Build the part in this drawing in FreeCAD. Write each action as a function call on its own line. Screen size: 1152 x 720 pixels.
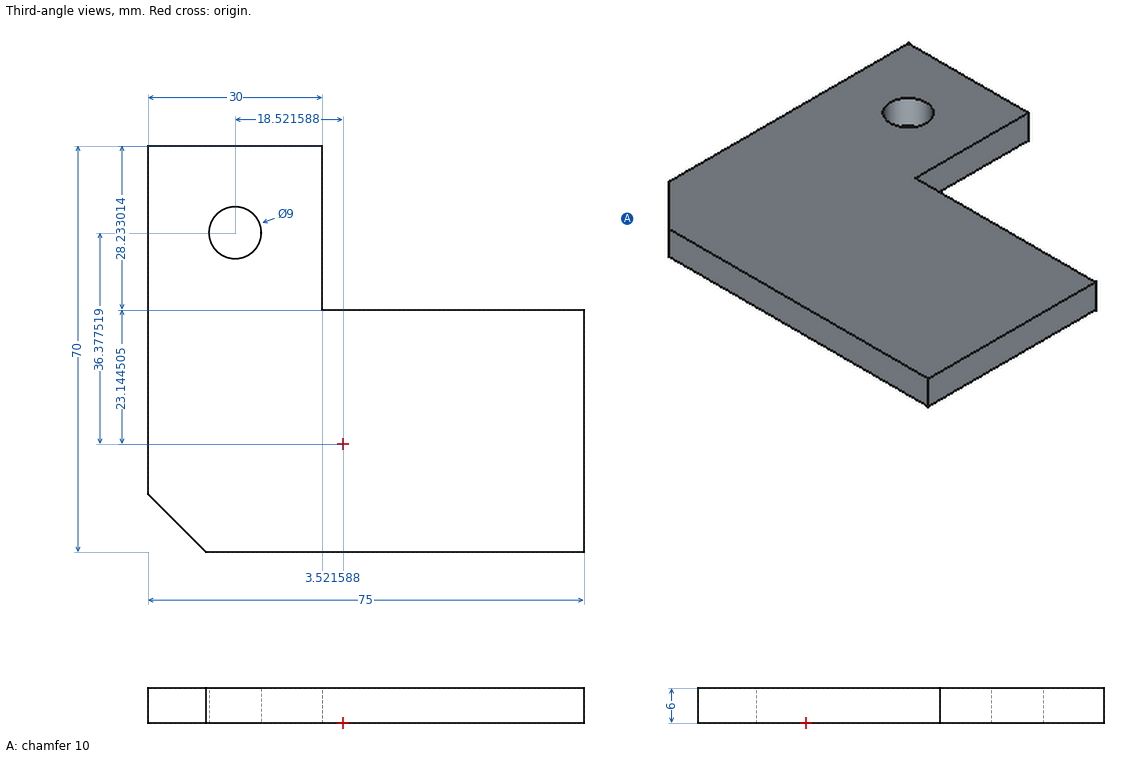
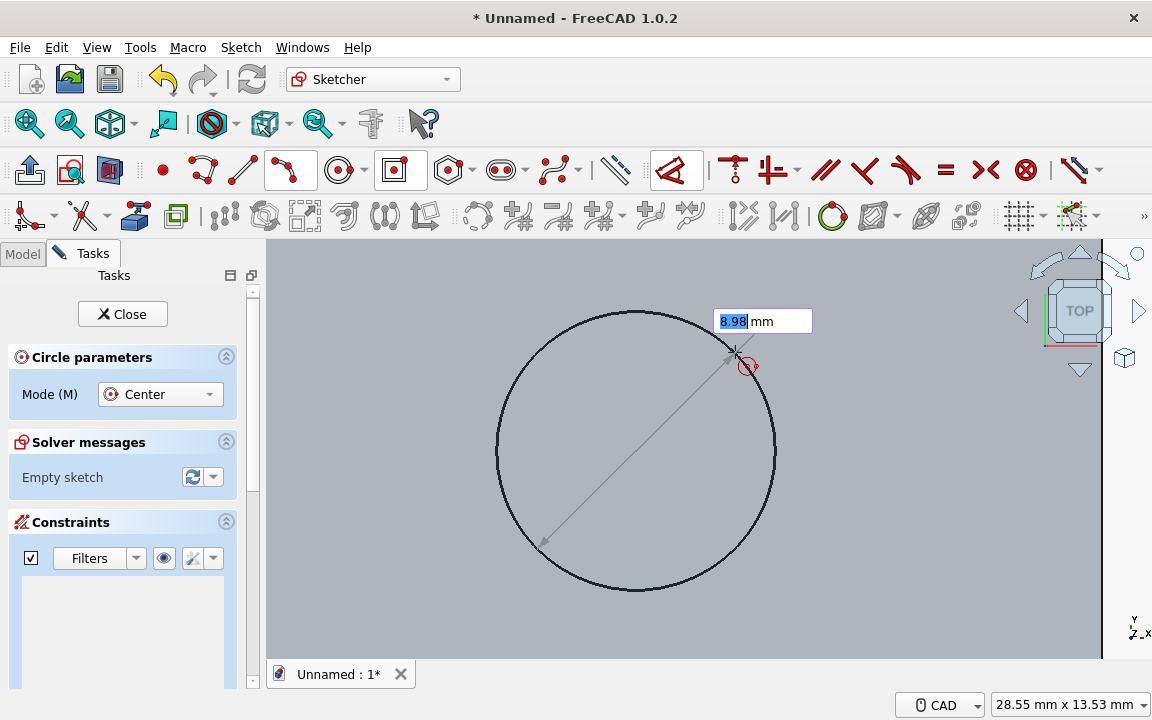
text(9)
key(Return)
key(Escape)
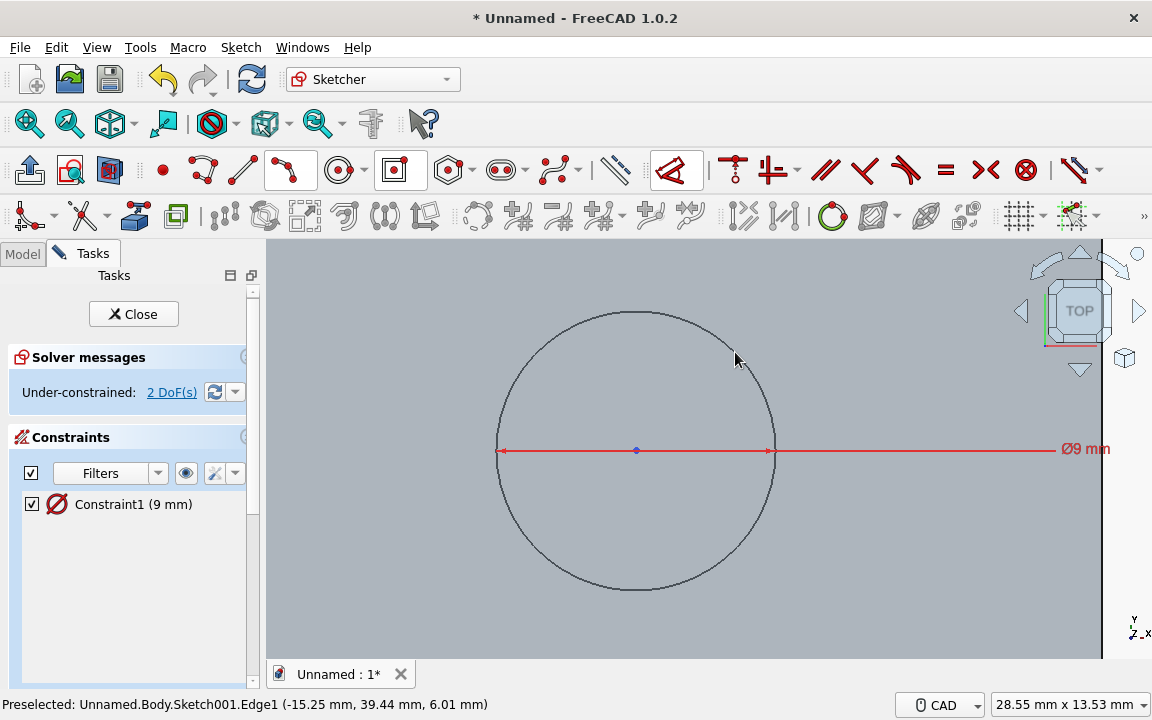
click(636, 451)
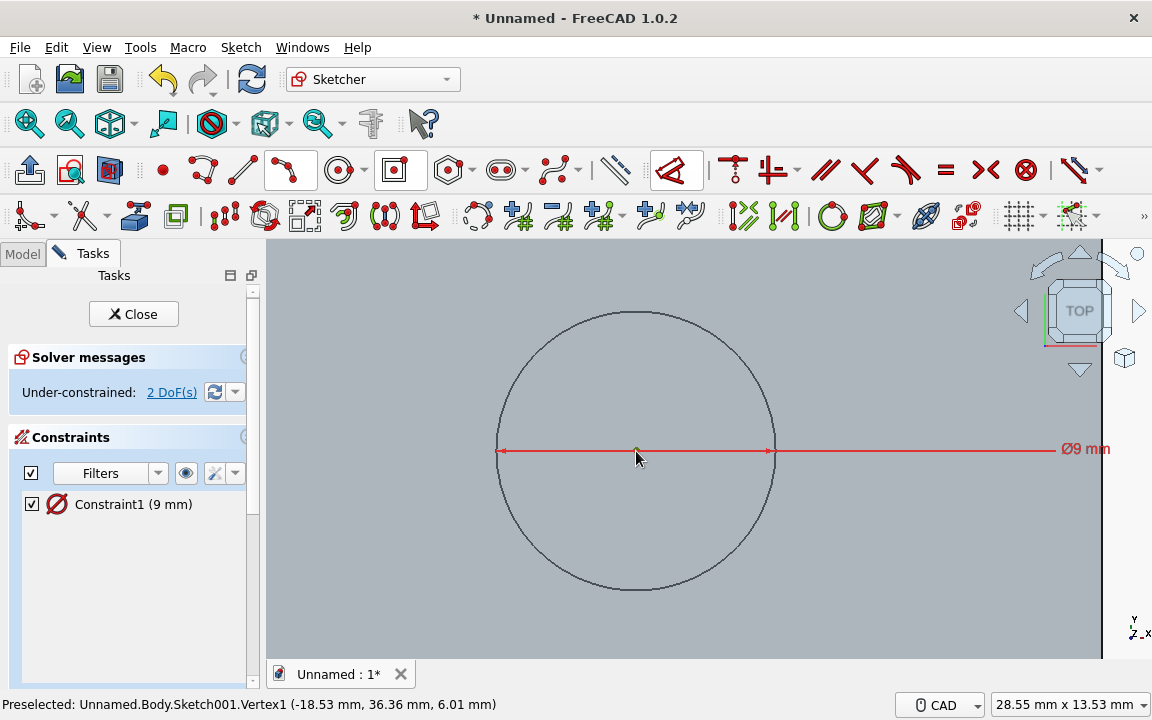
click(698, 170)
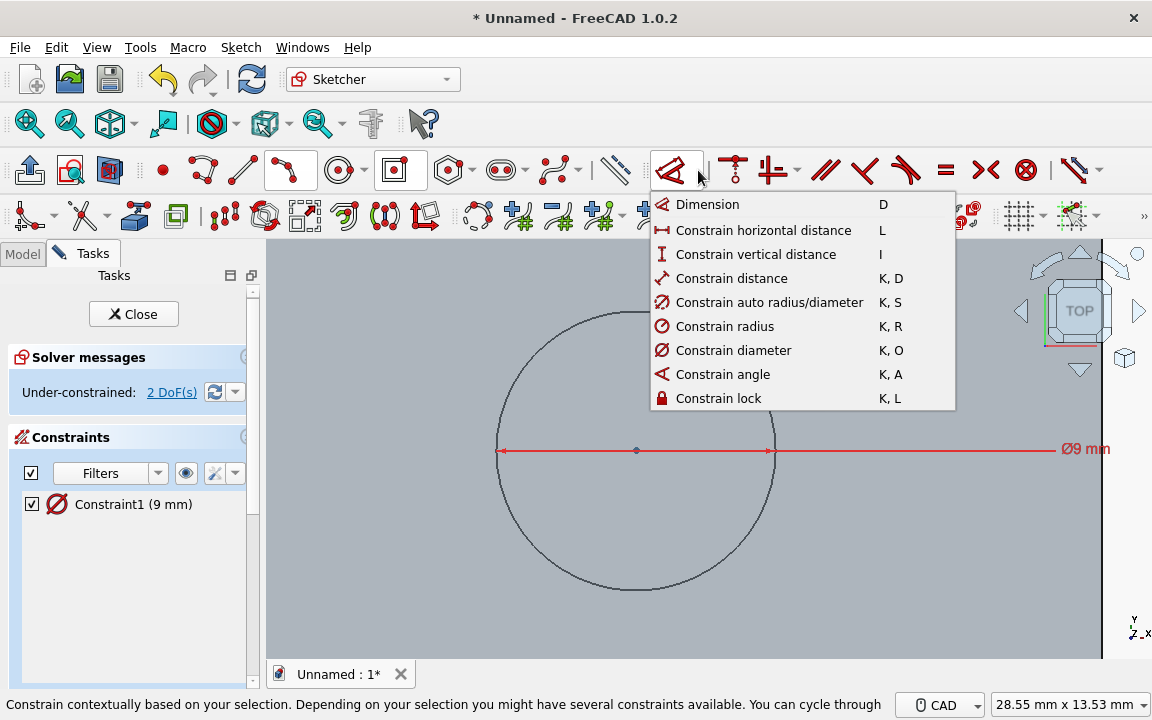
click(803, 230)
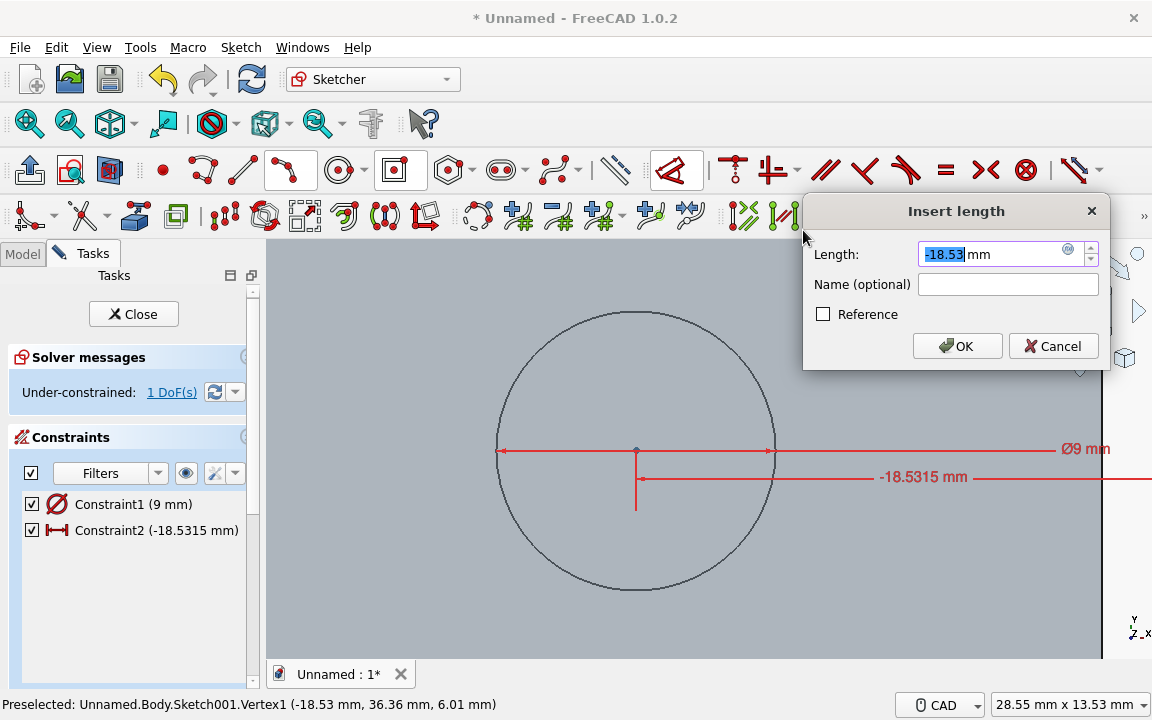
text(-18.521588)
key(Return)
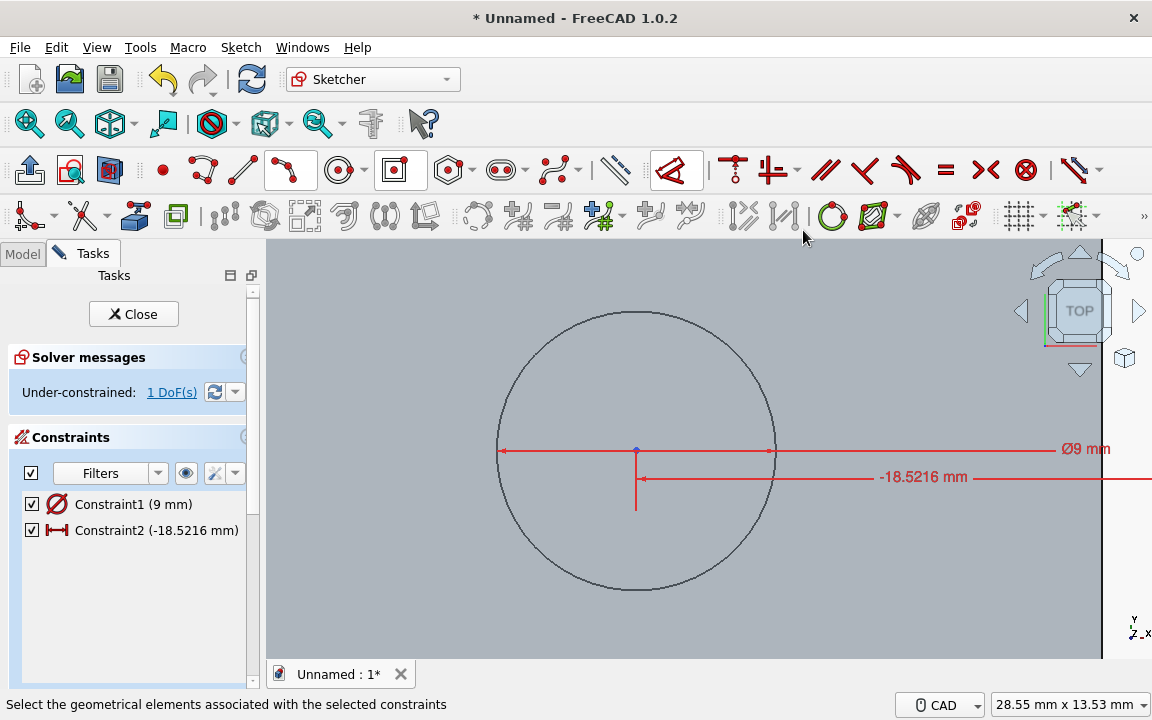
click(636, 451)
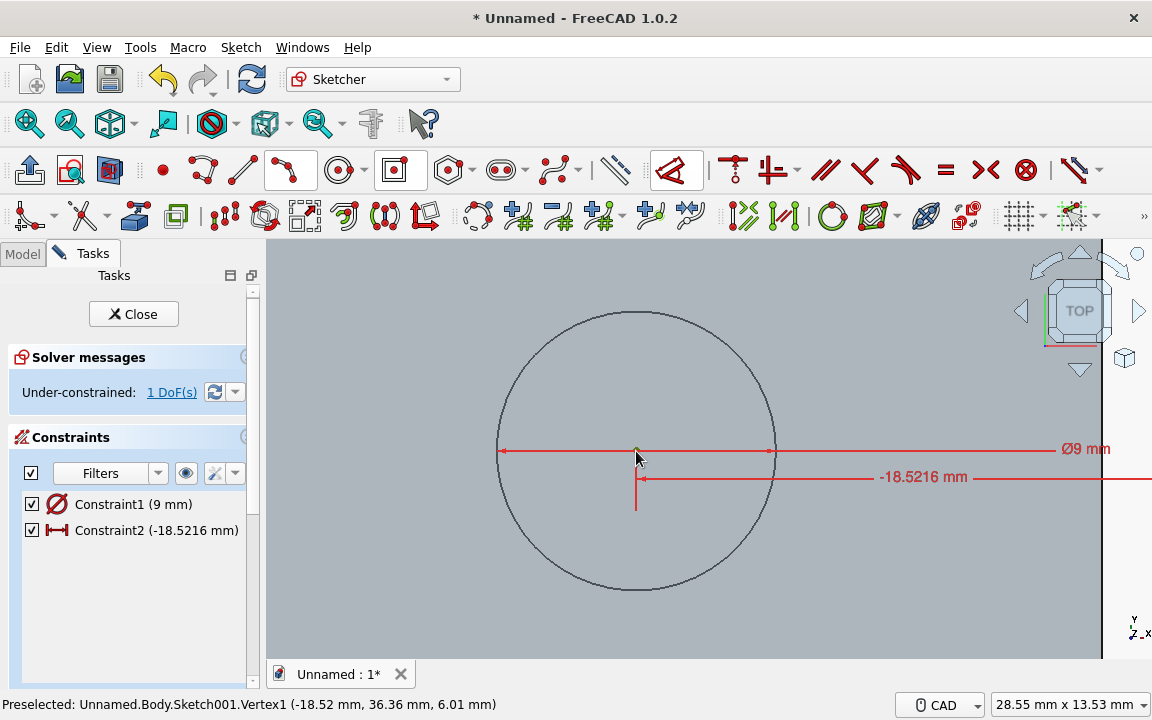
click(698, 170)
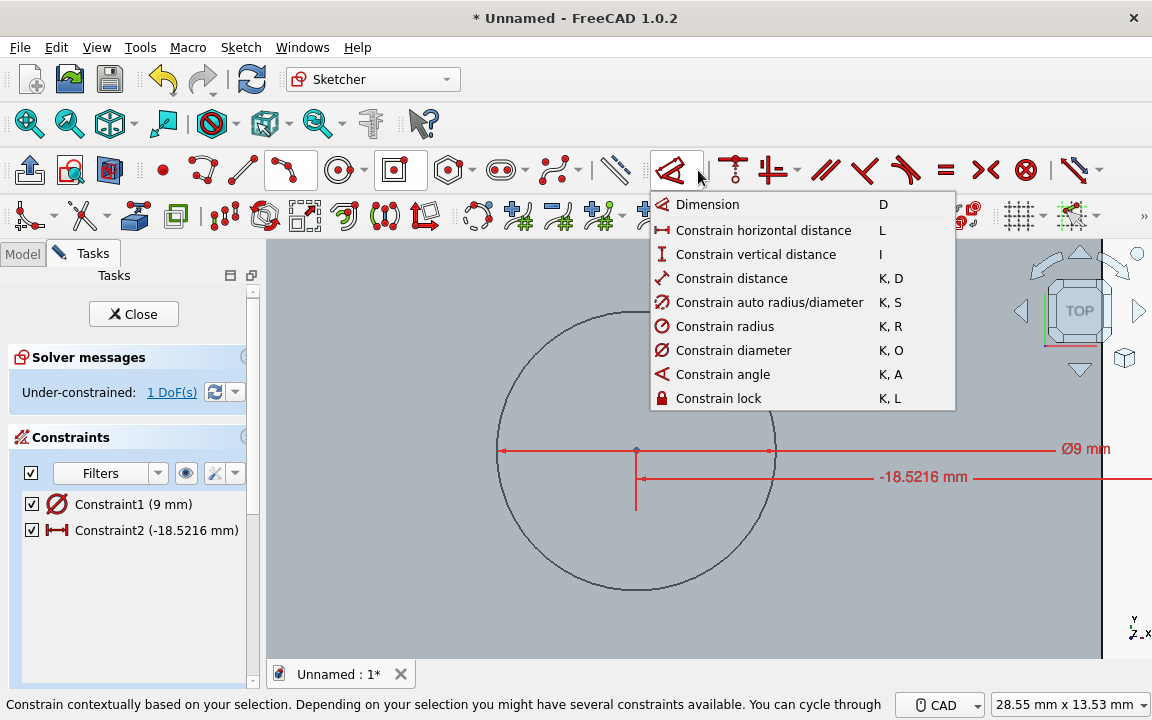
click(803, 254)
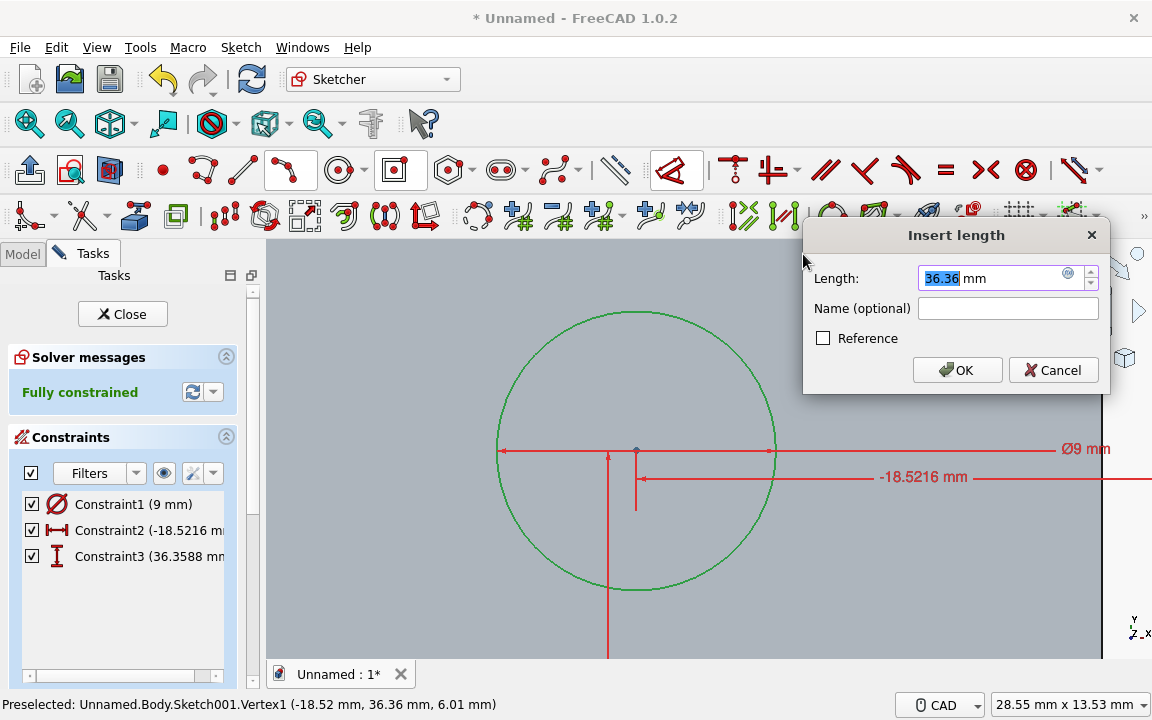
text(36.377519)
key(Return)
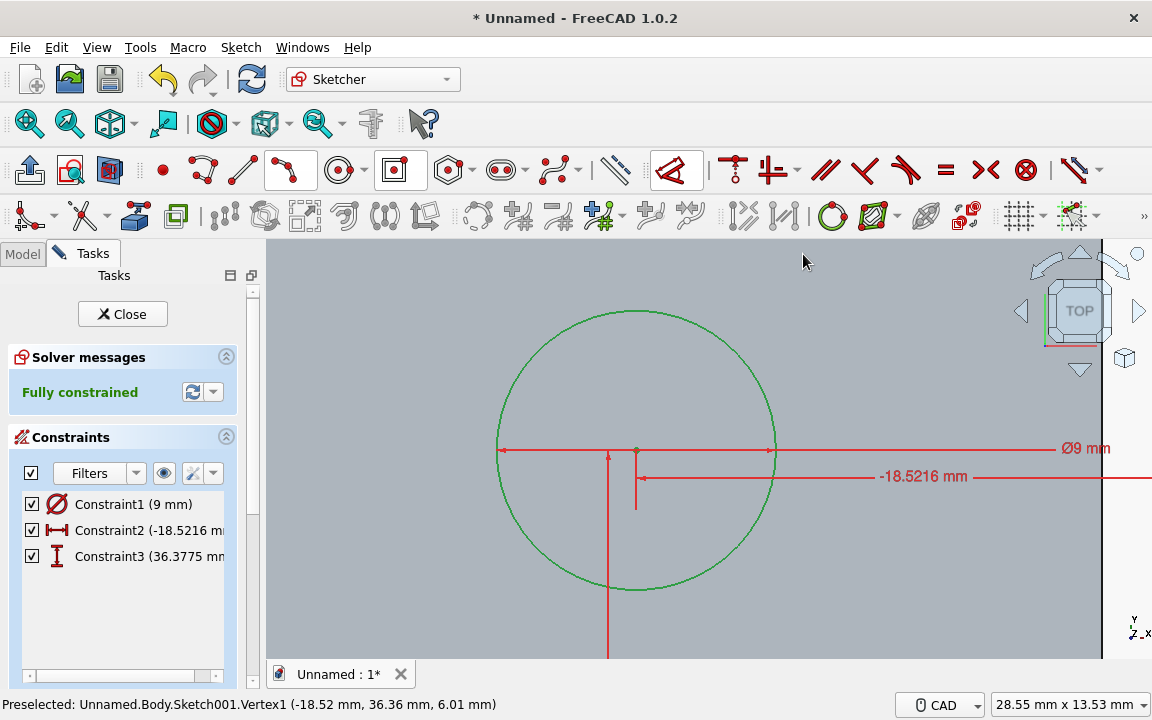
click(123, 314)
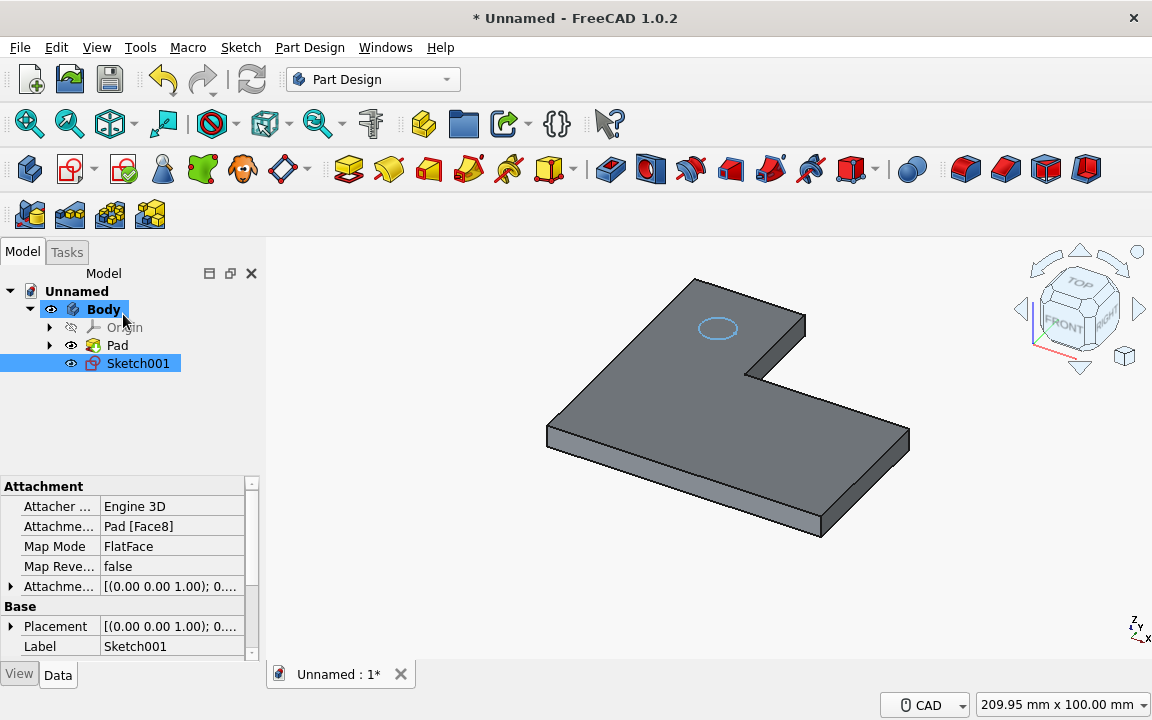
click(612, 170)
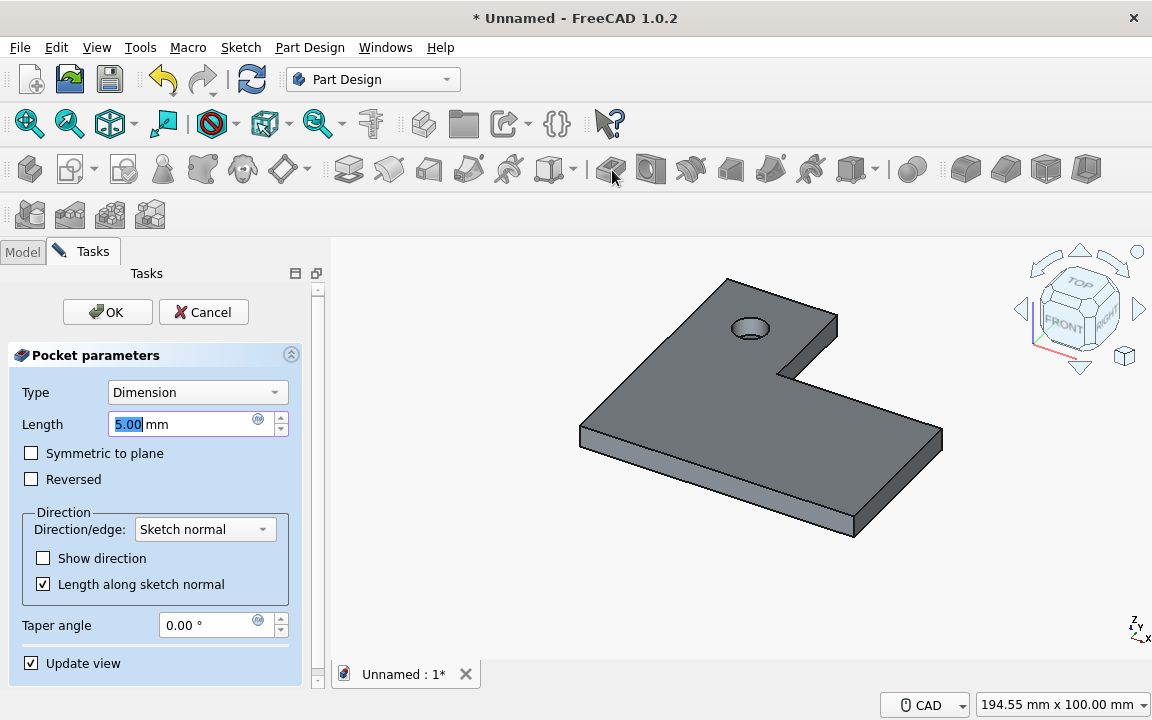
click(198, 392)